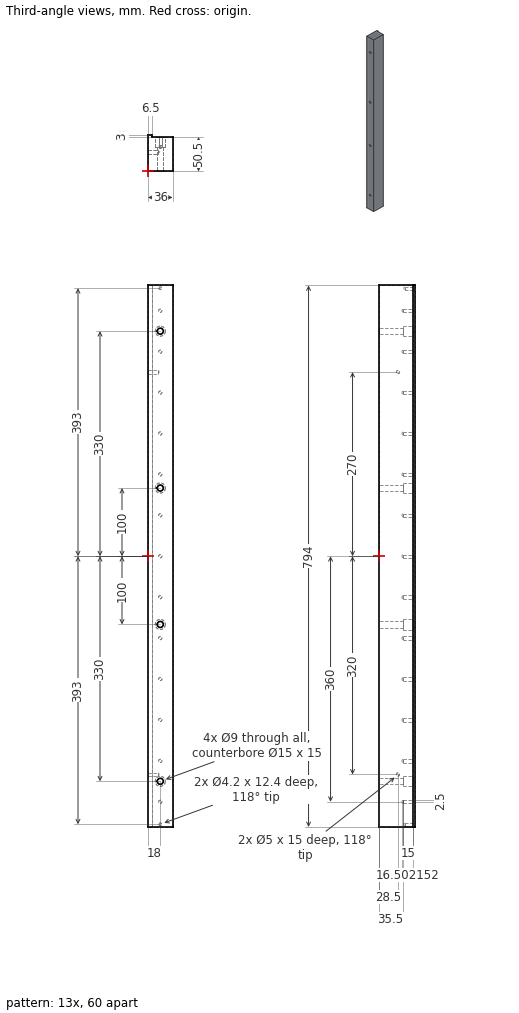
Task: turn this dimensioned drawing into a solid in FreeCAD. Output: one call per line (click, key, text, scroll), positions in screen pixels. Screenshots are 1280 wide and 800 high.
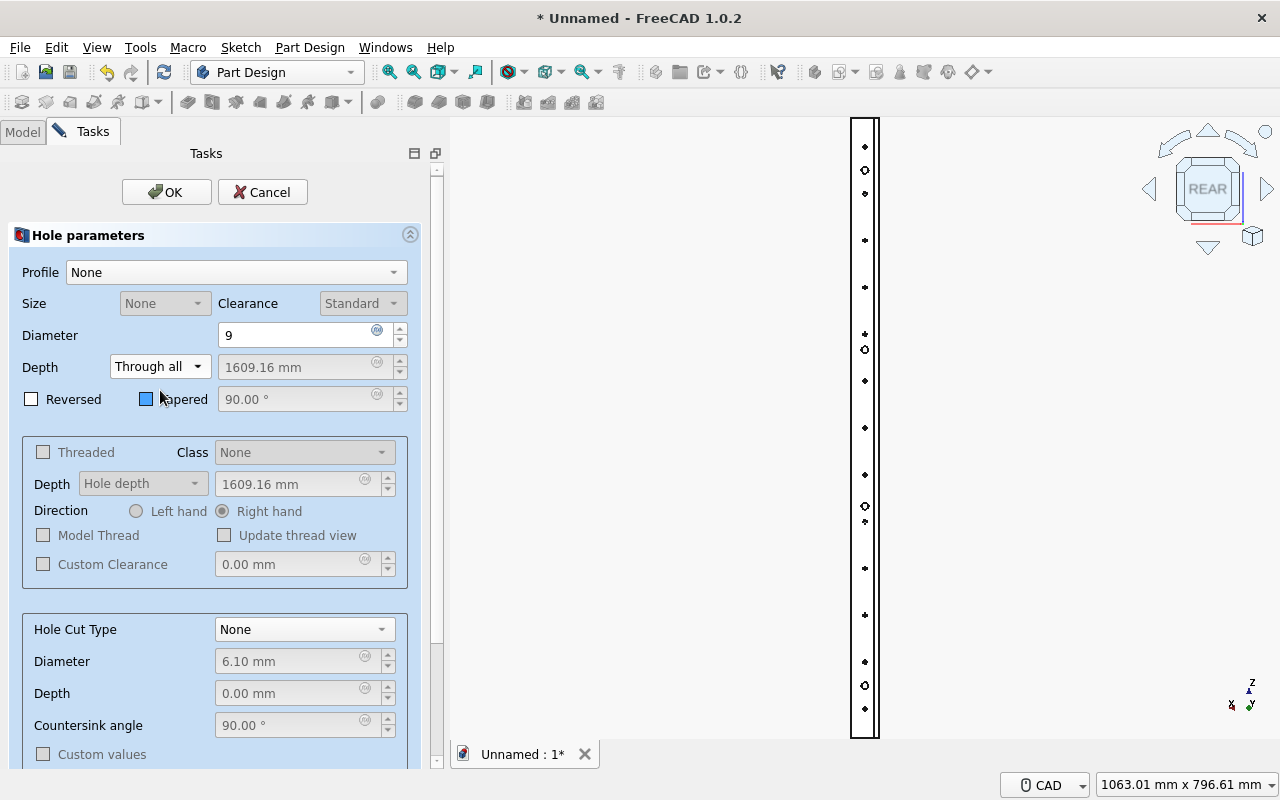
click(306, 630)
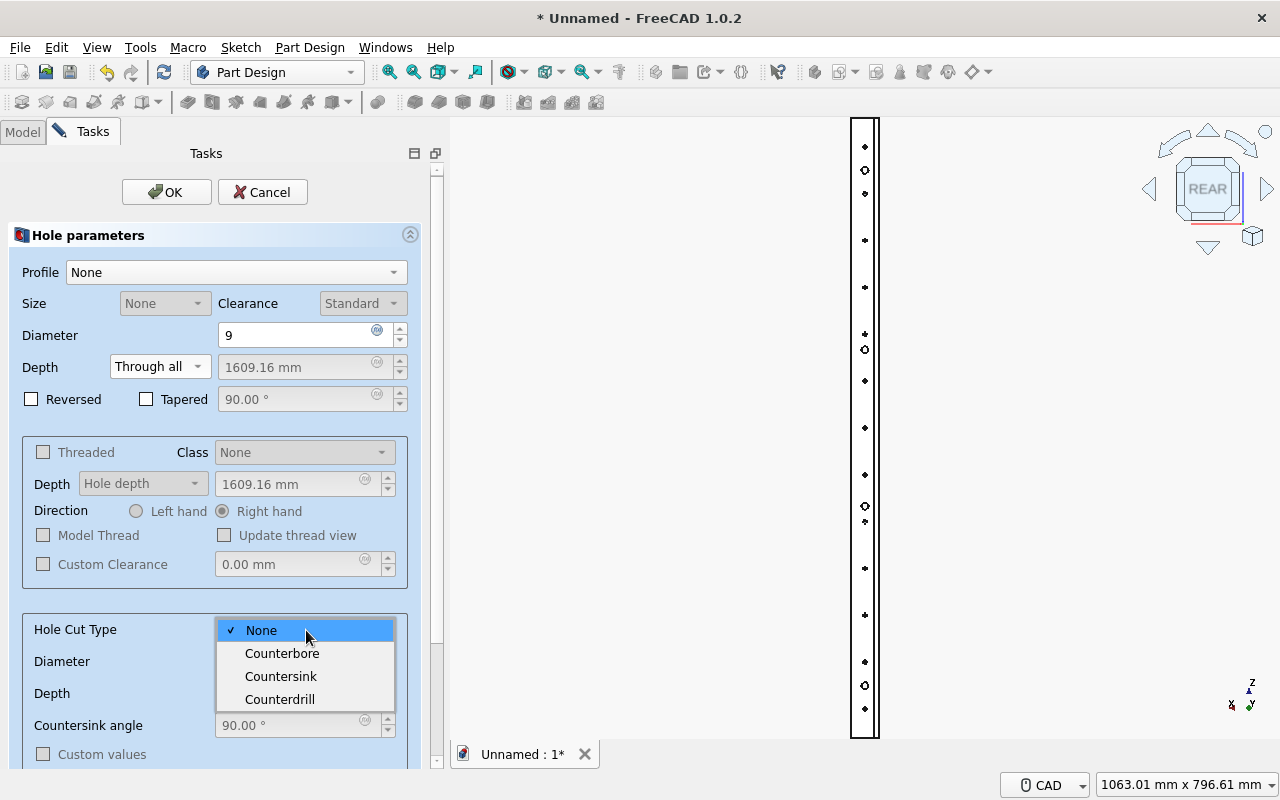
click(304, 654)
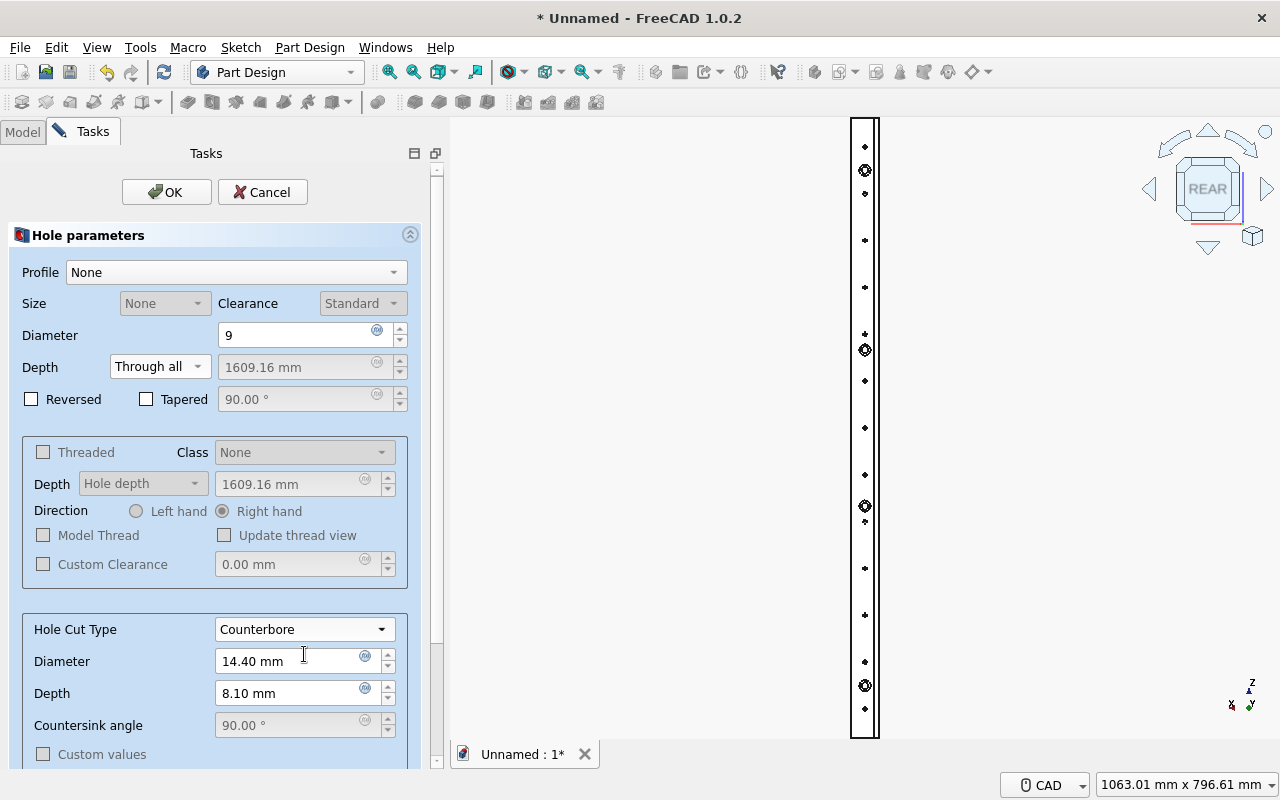
triple_click(298, 661)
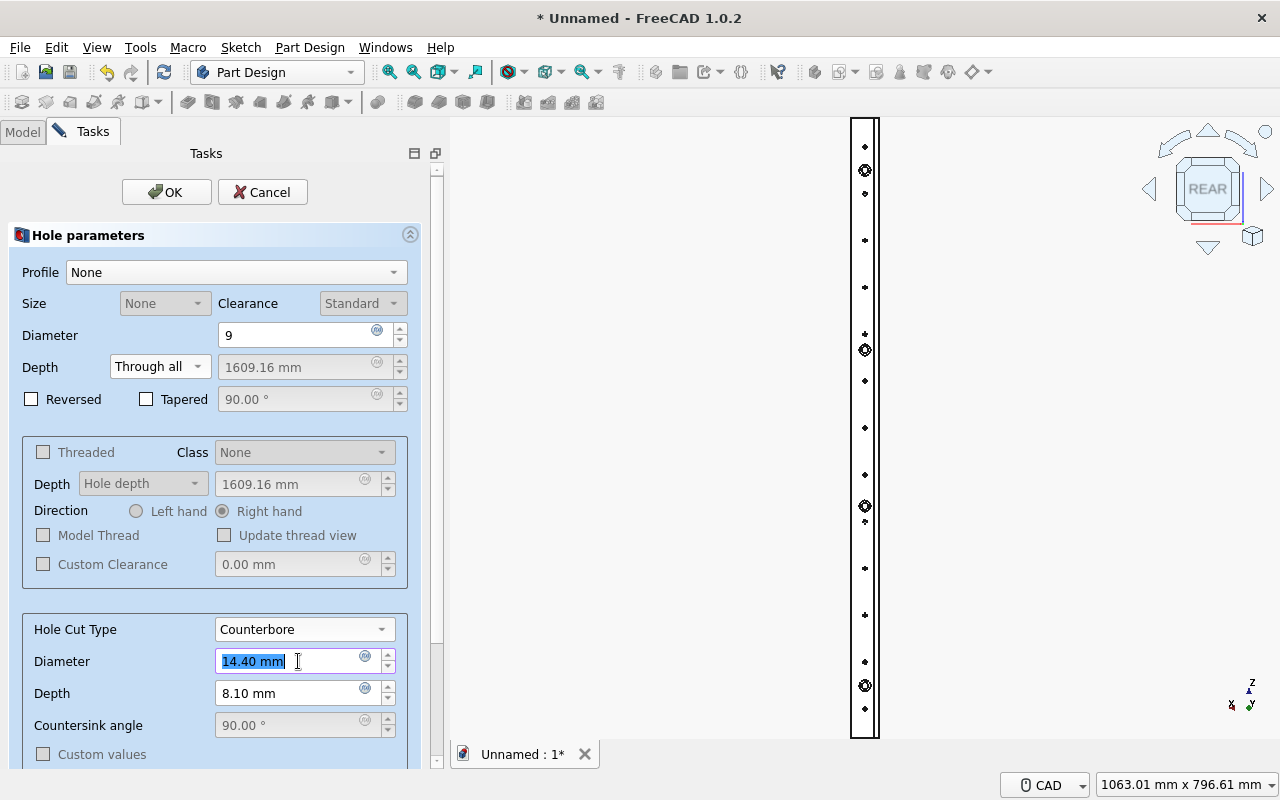
text(15)
key(Tab)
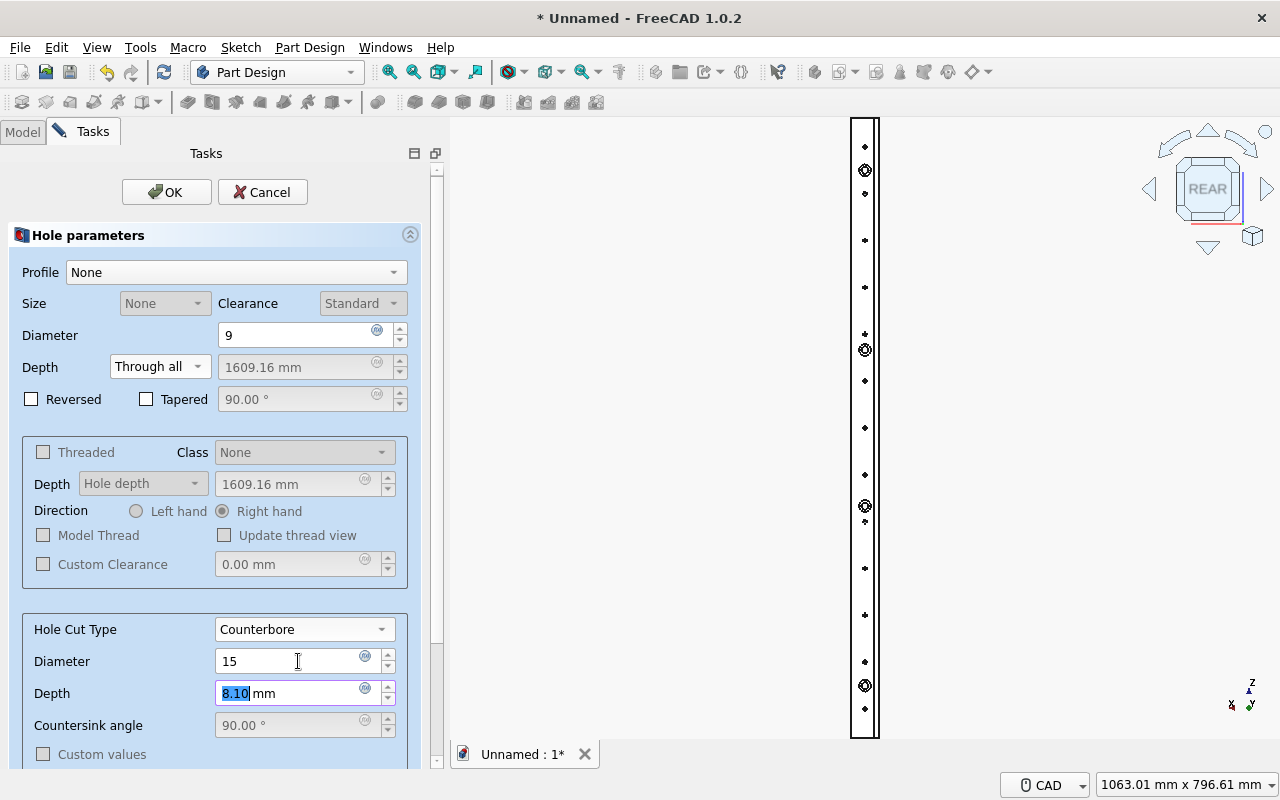
text(15)
key(Tab)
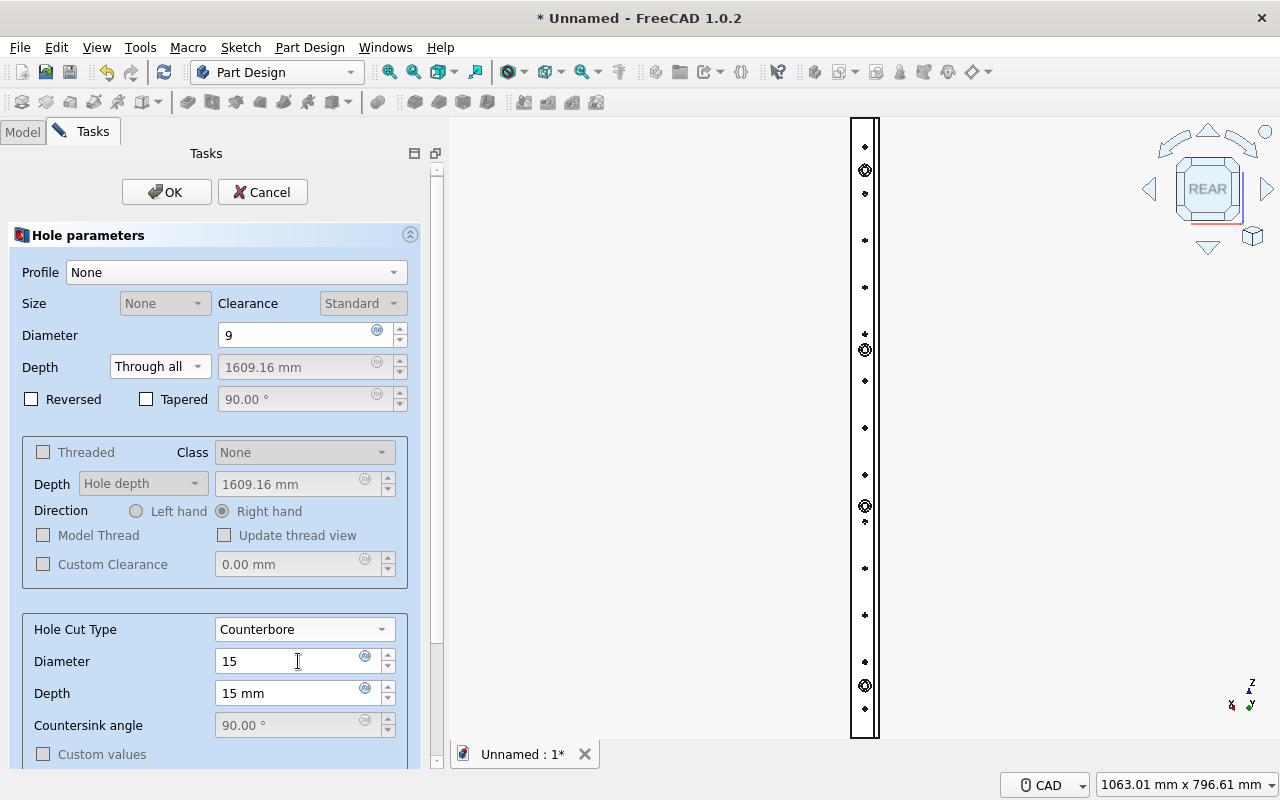
click(167, 192)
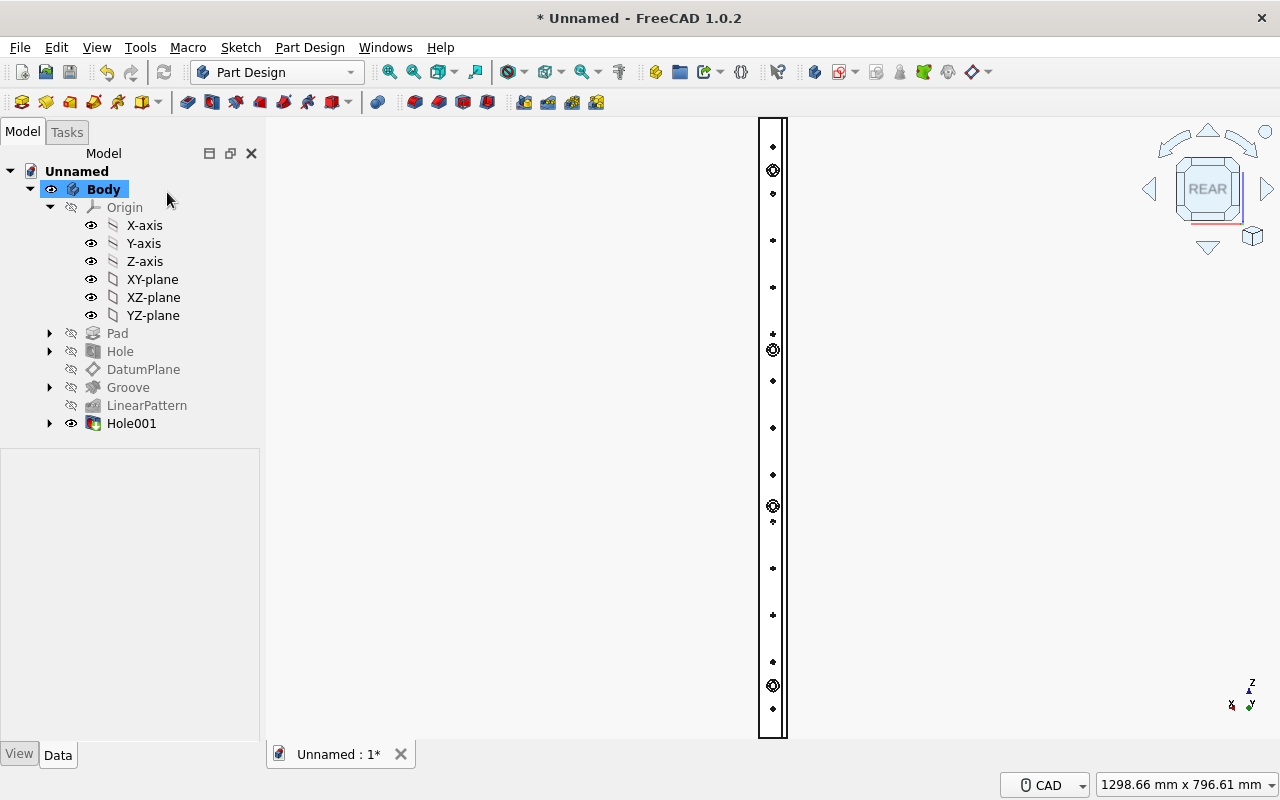
click(770, 604)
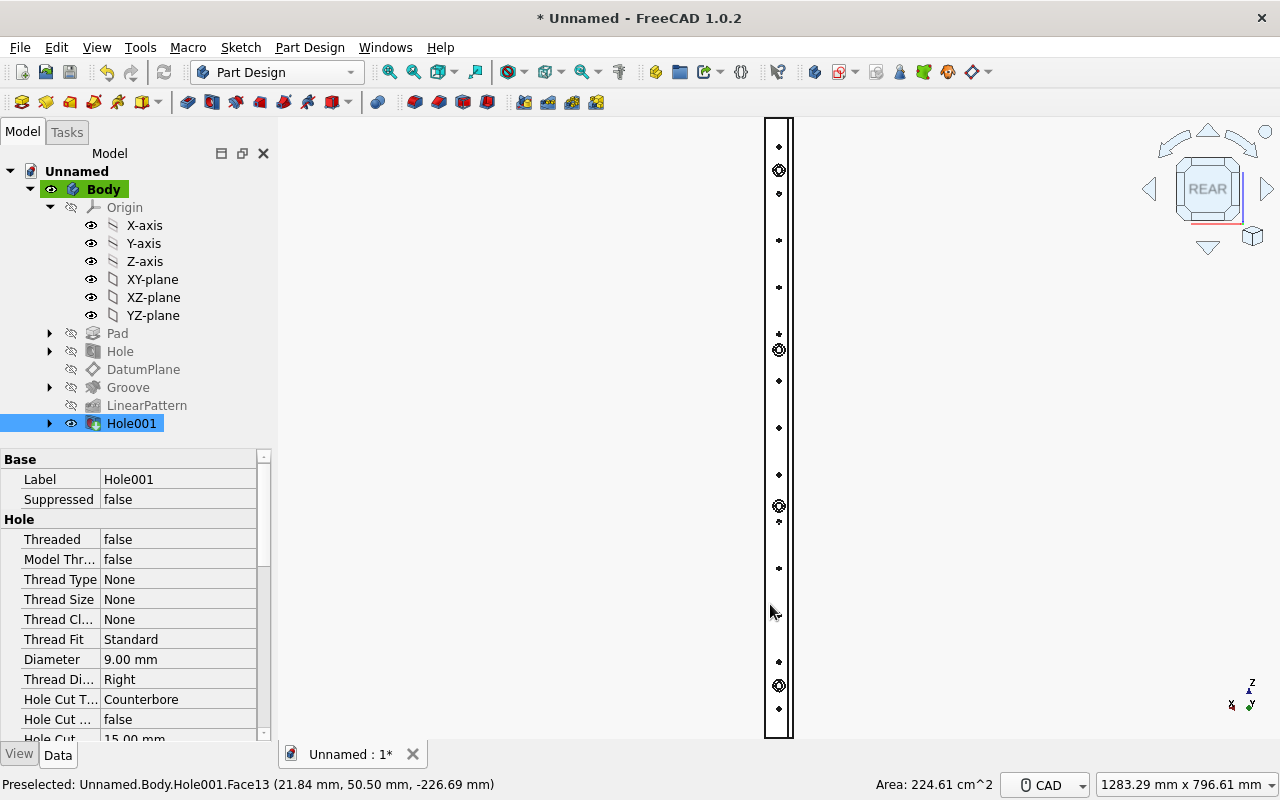
click(840, 72)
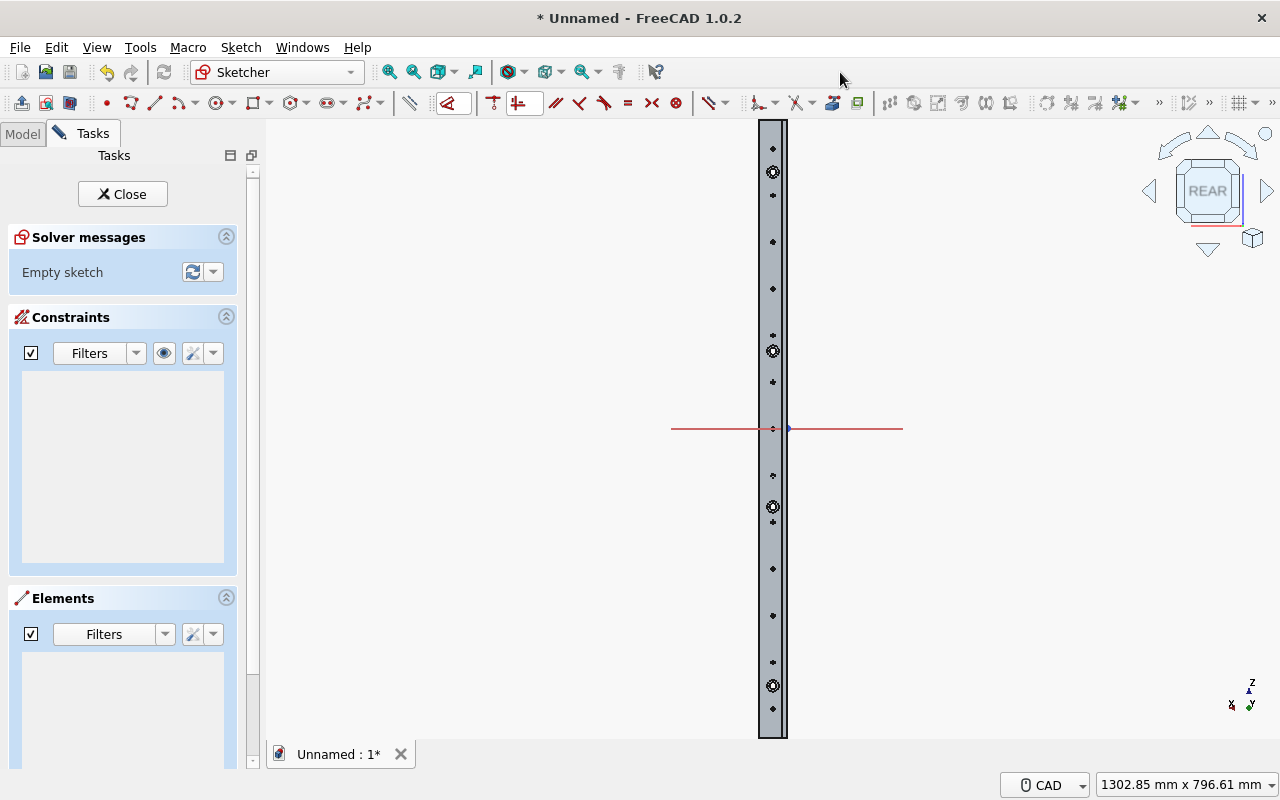
click(70, 104)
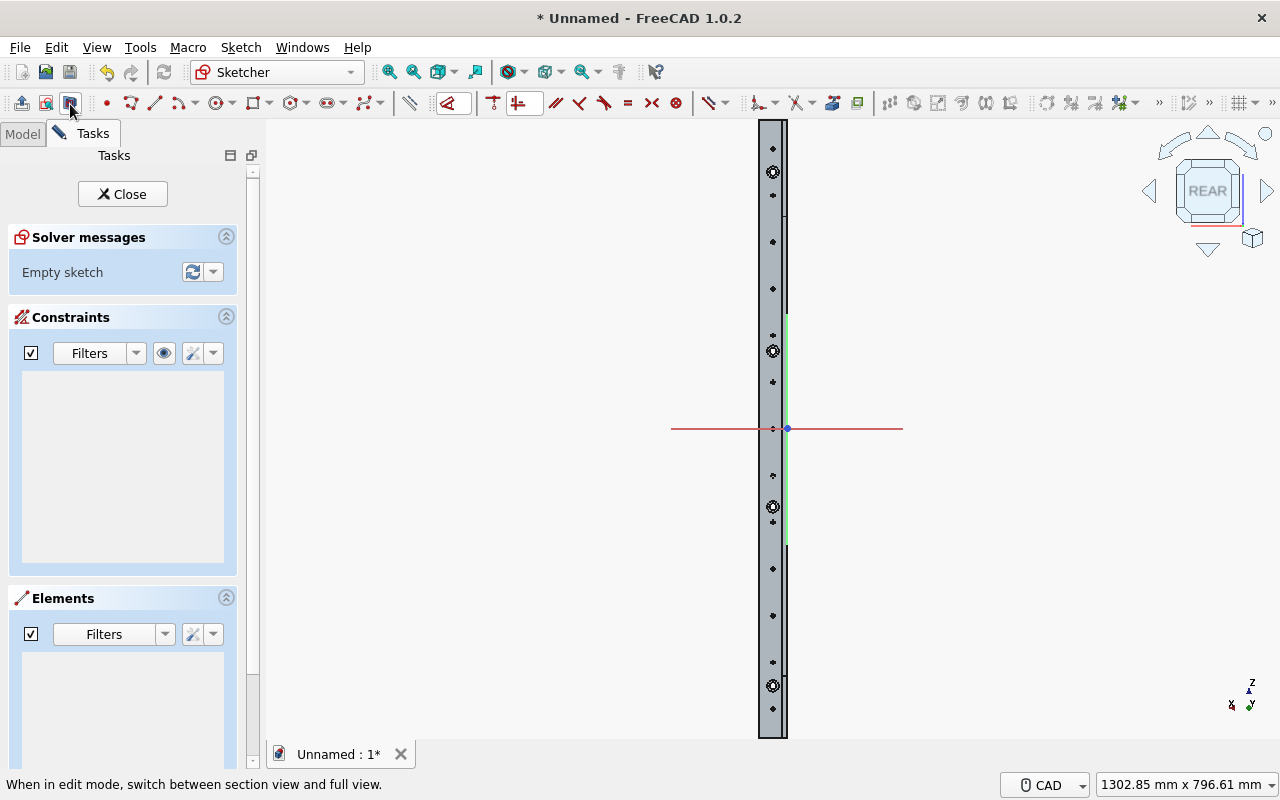
scroll(553, 429, down, 2)